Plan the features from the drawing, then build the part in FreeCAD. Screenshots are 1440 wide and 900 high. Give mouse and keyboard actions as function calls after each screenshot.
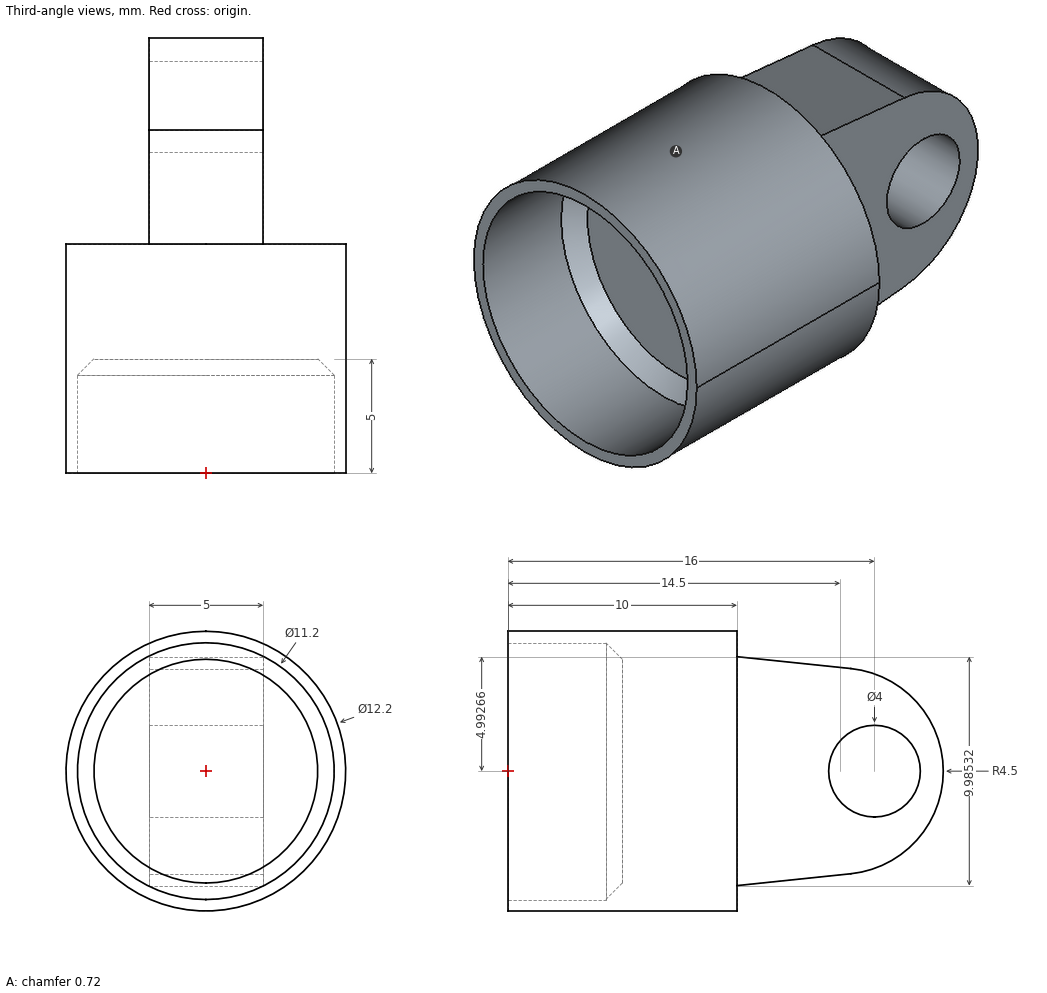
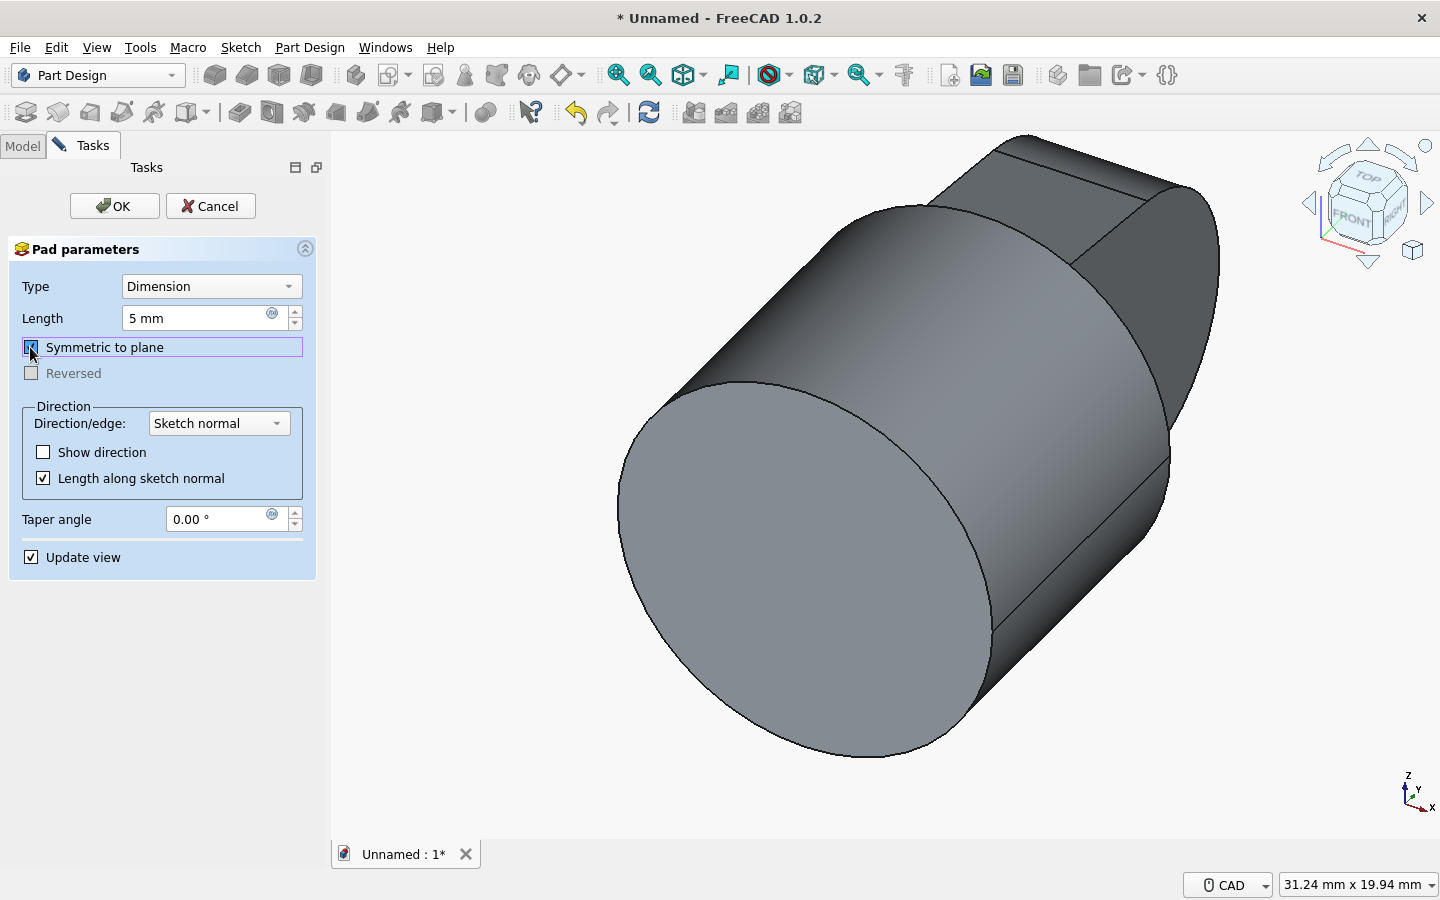
click(115, 206)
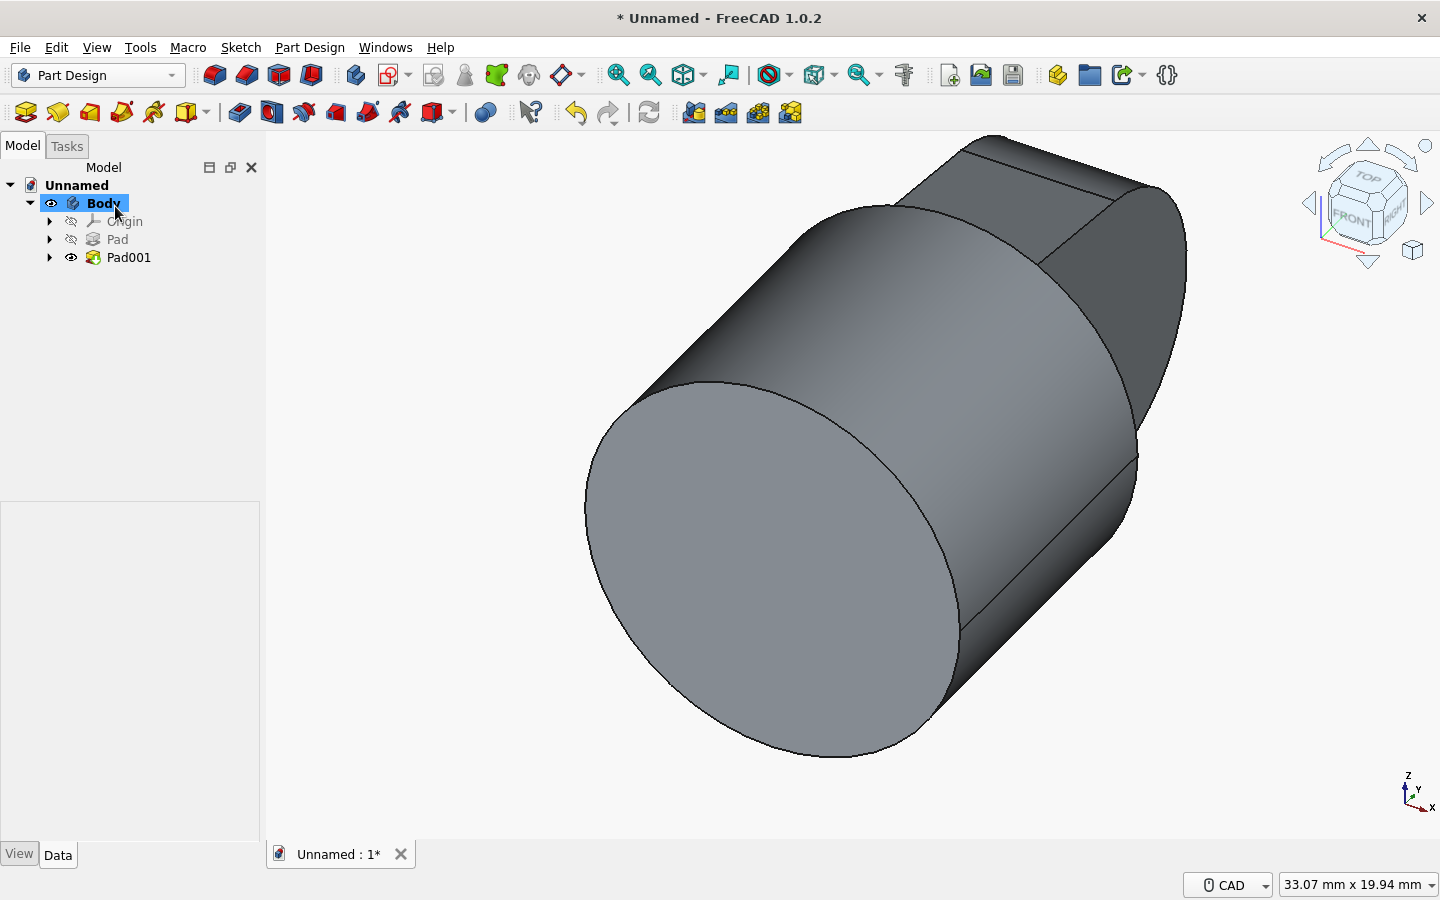
key(v)
key(f)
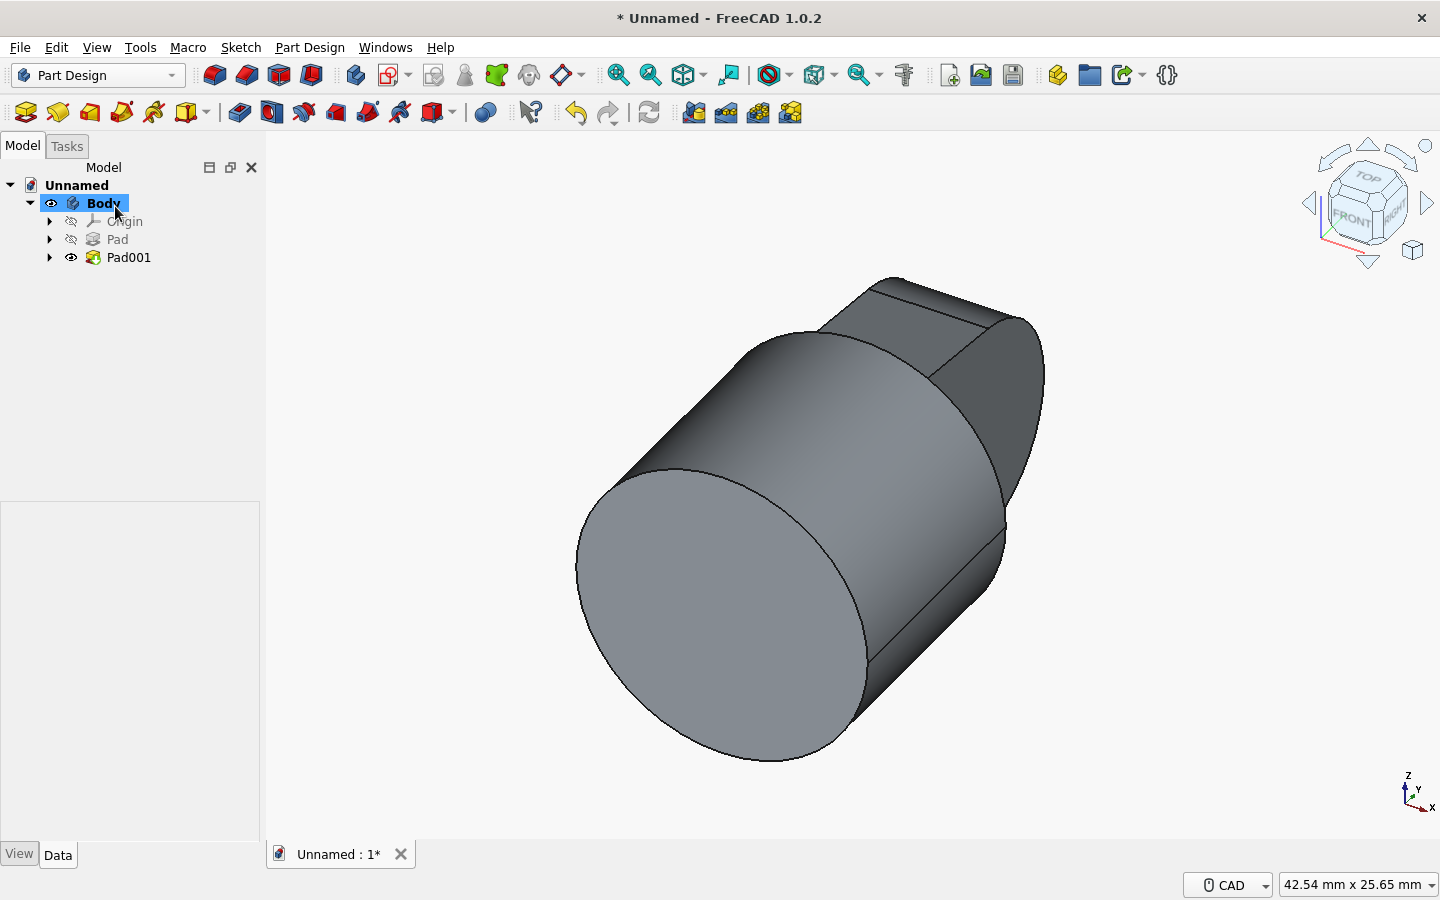
click(1000, 418)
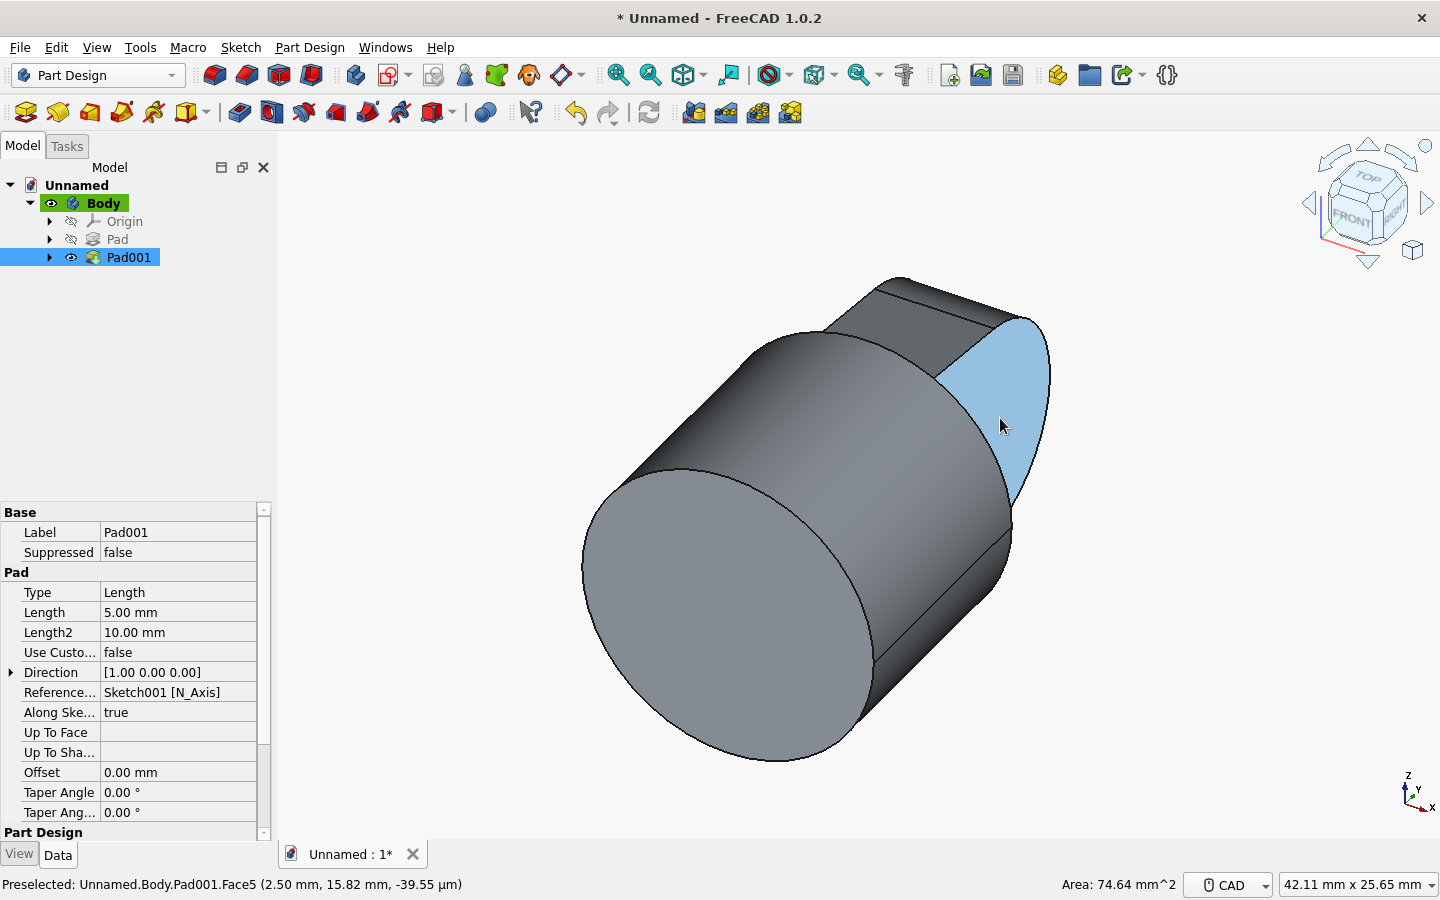
click(388, 76)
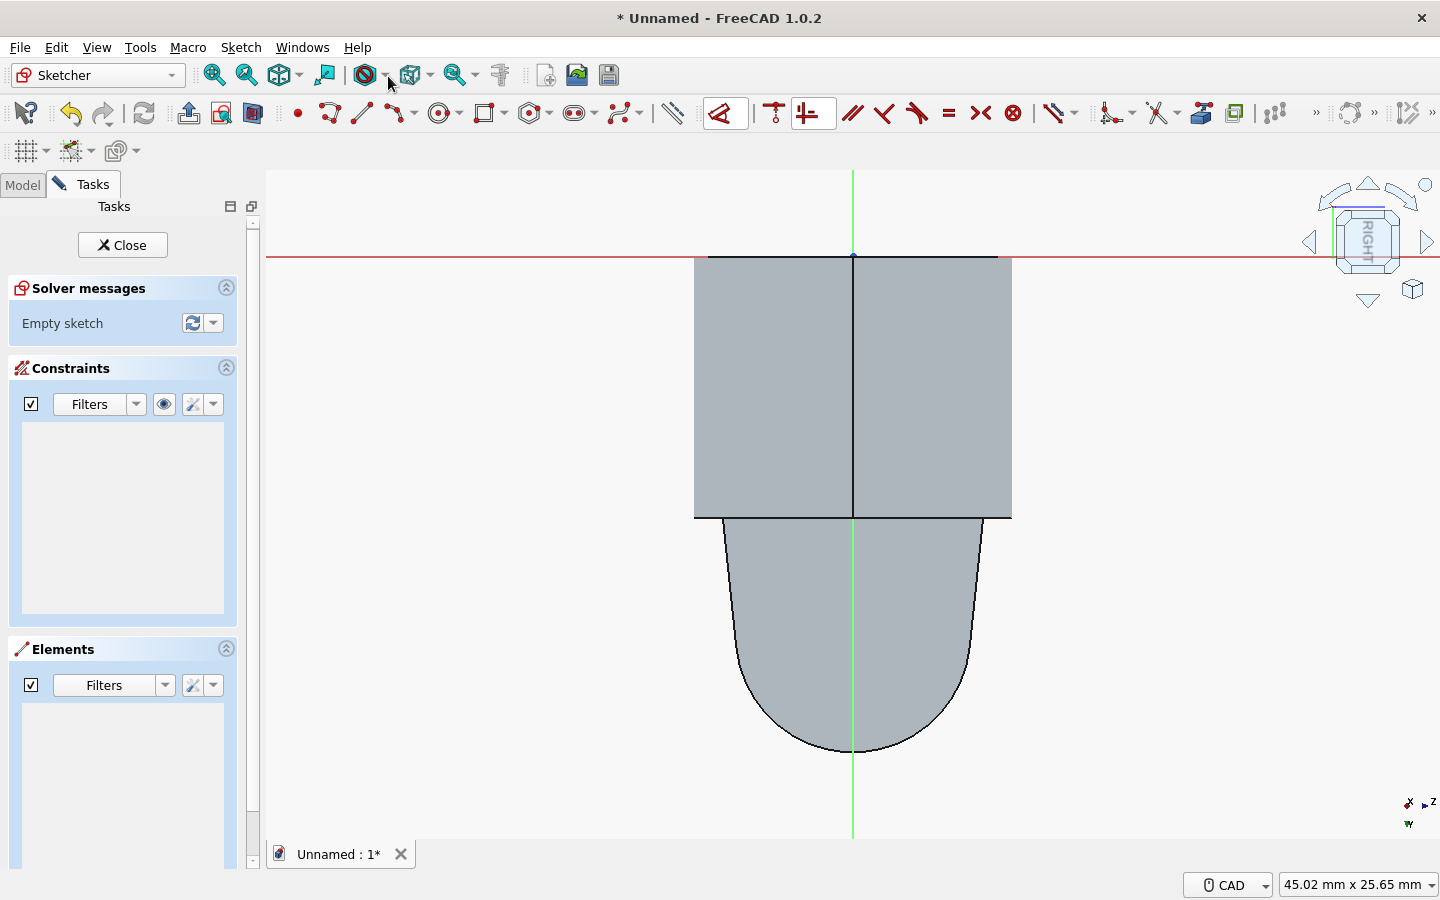
scroll(875, 730, up, 7)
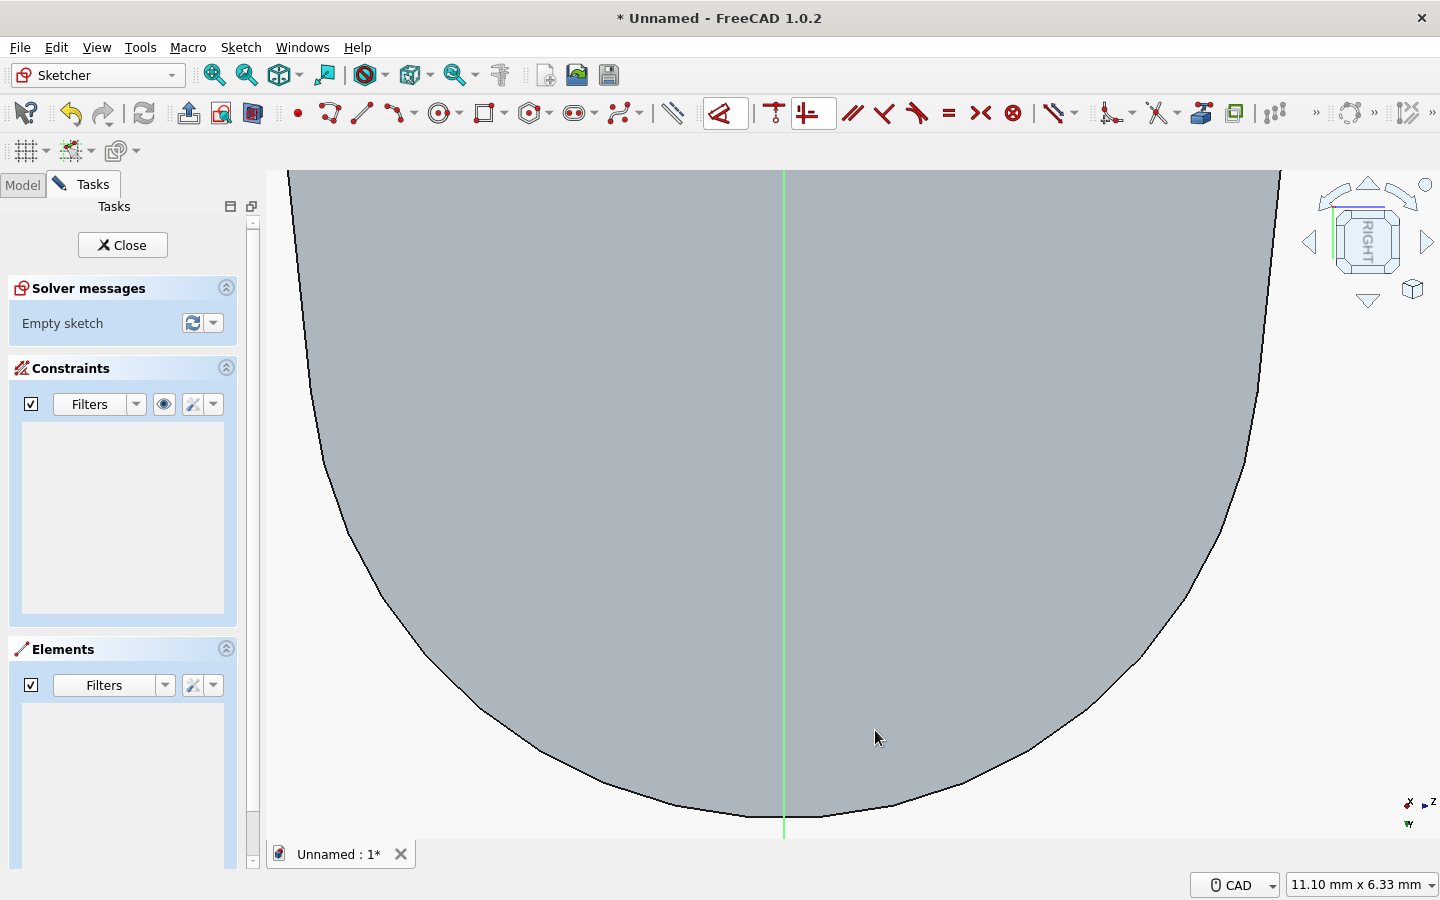
key(g)
key(c)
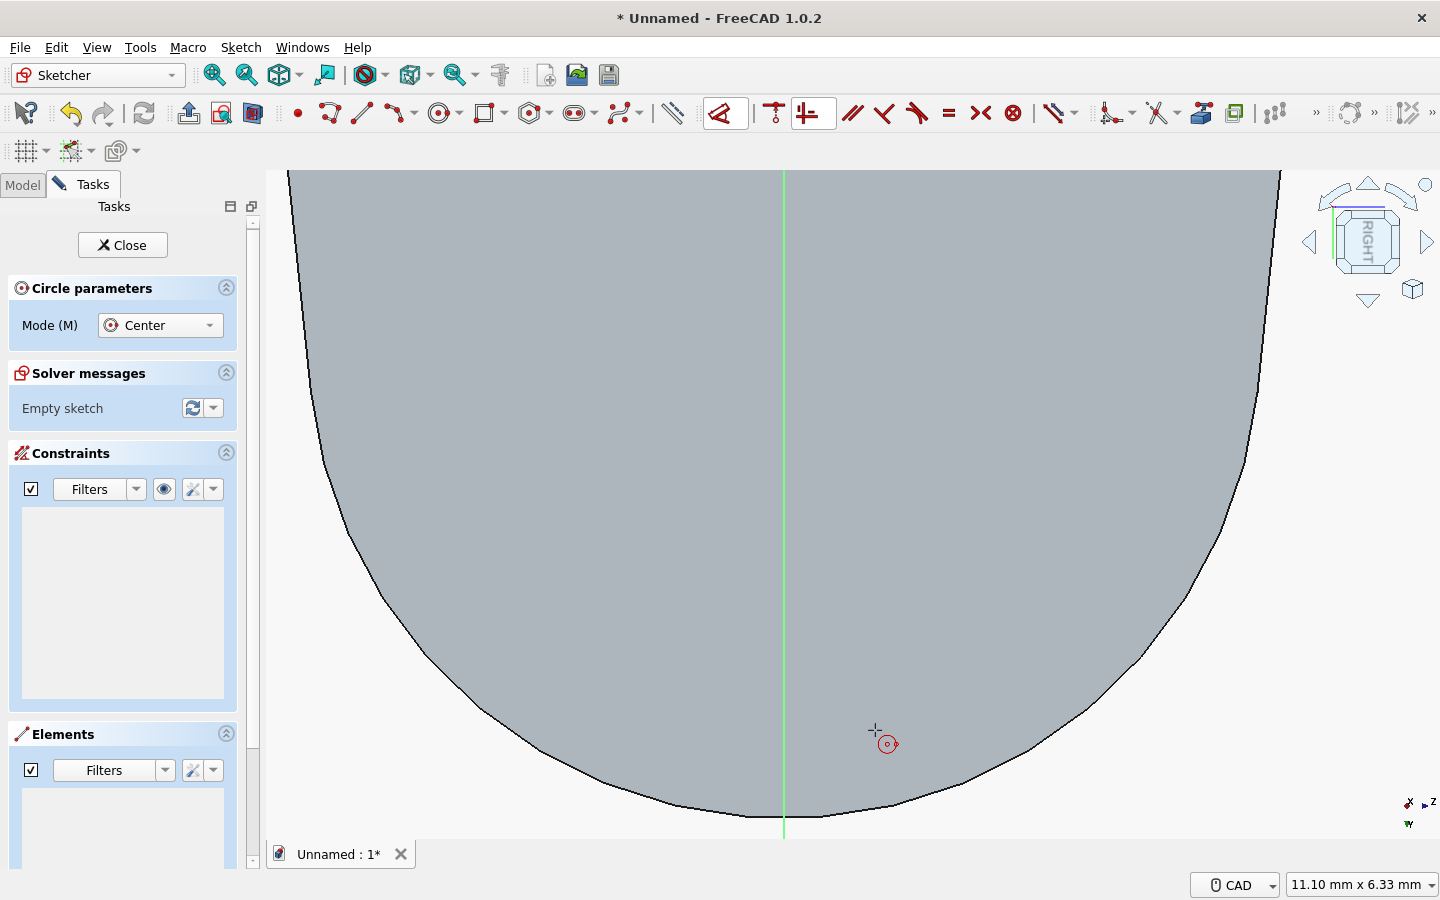
click(784, 501)
click(934, 352)
key(Escape)